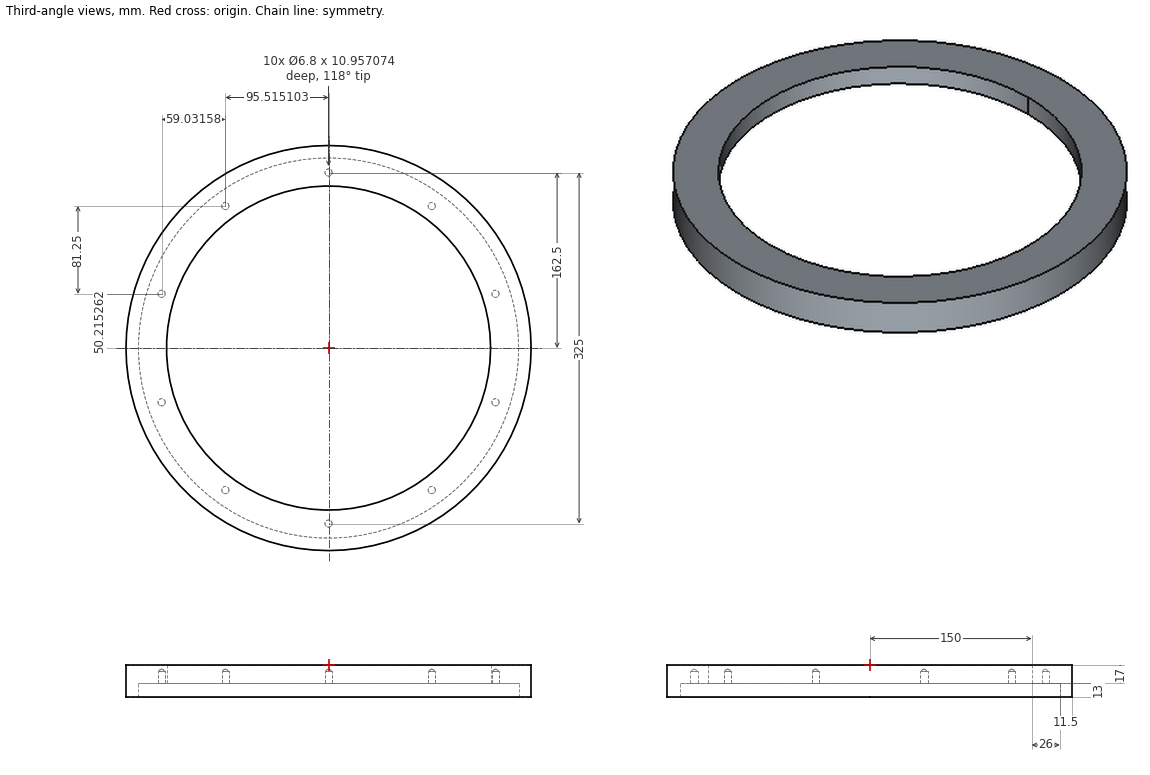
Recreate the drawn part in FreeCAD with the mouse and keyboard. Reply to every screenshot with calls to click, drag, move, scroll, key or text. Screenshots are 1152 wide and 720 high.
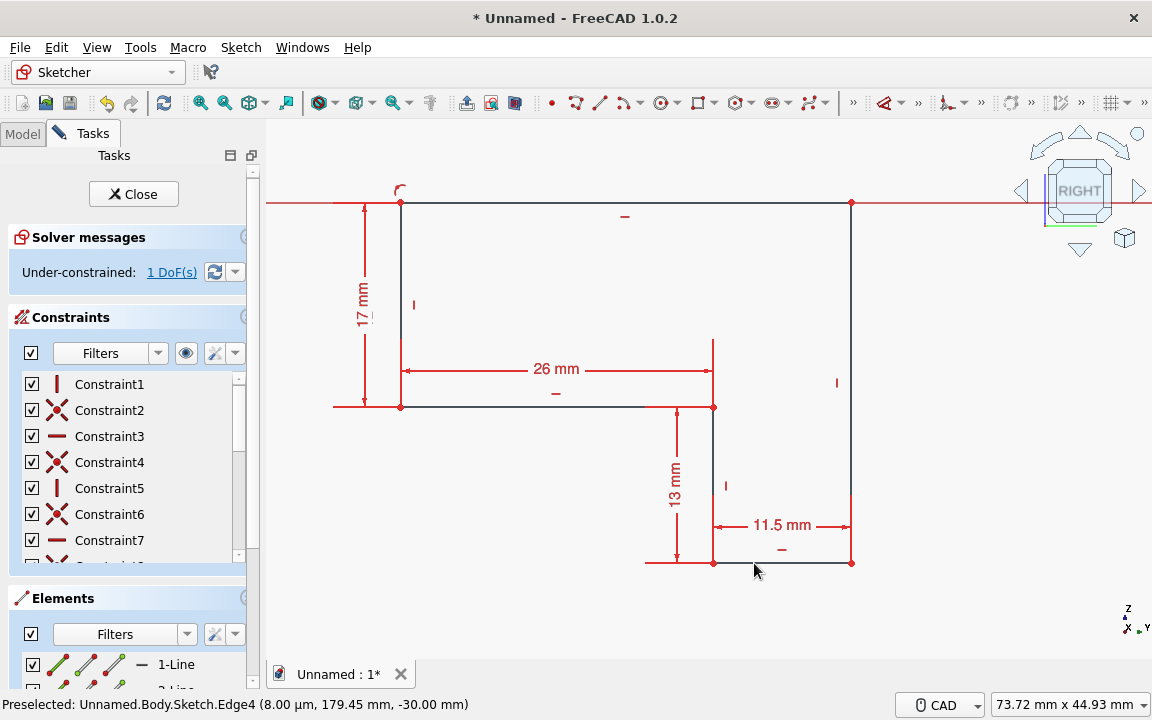
click(401, 203)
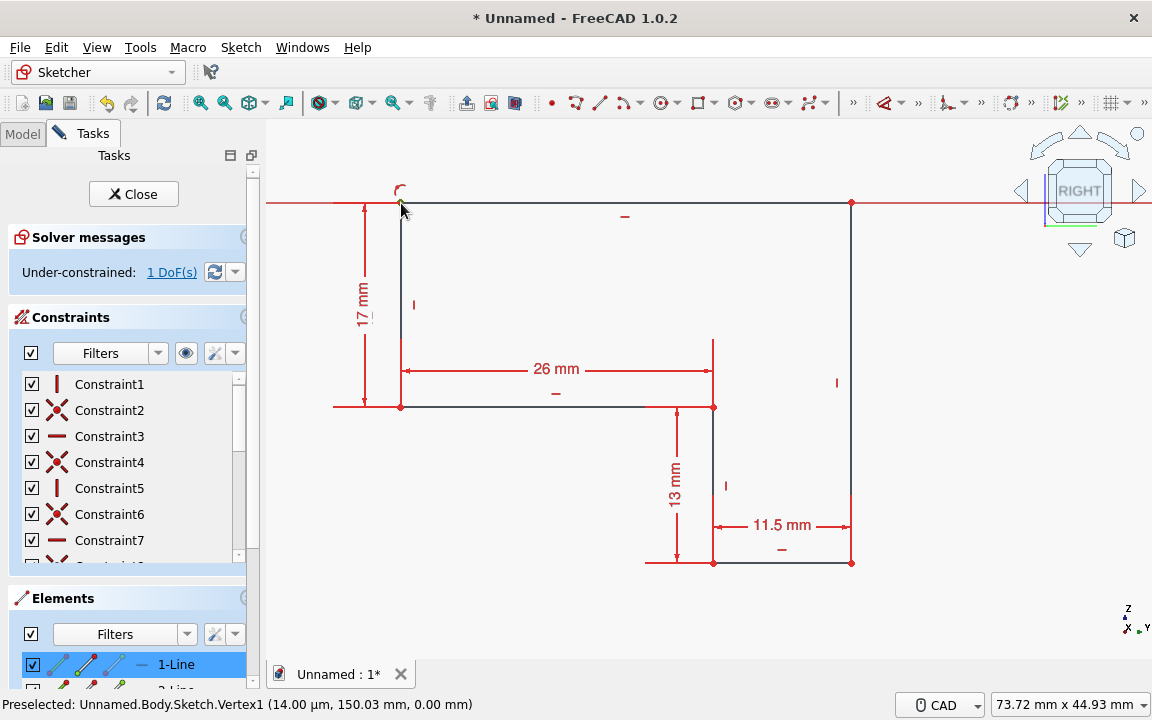
key(l)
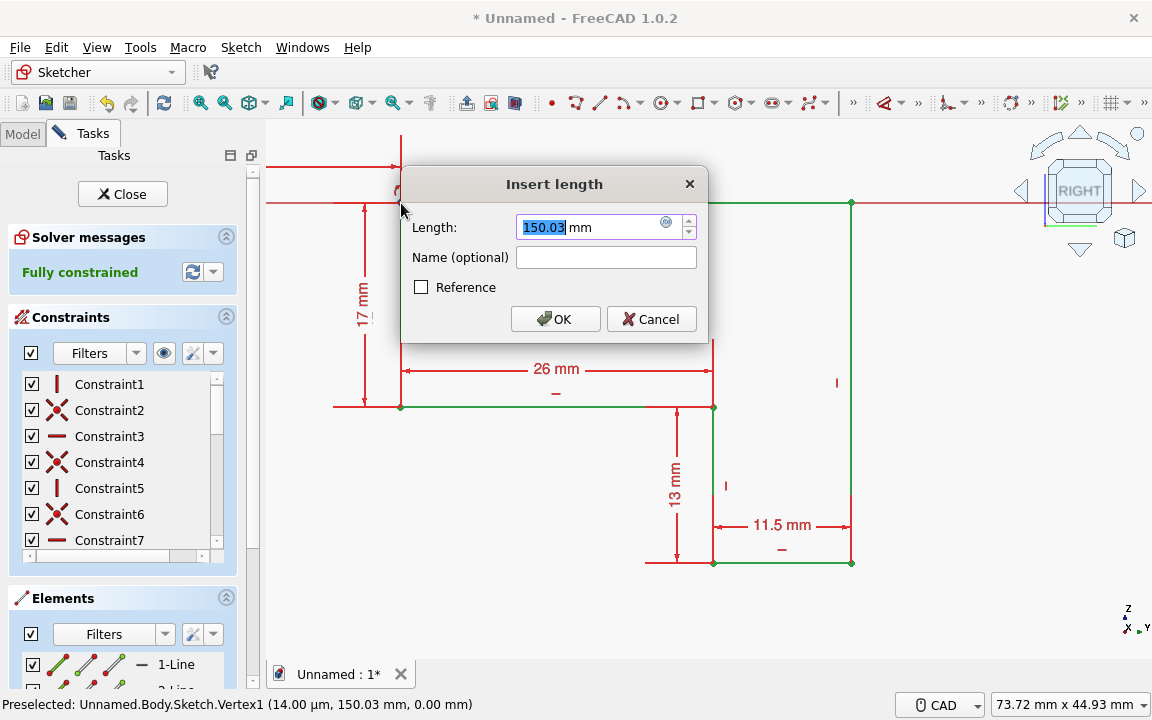
text(150)
key(Return)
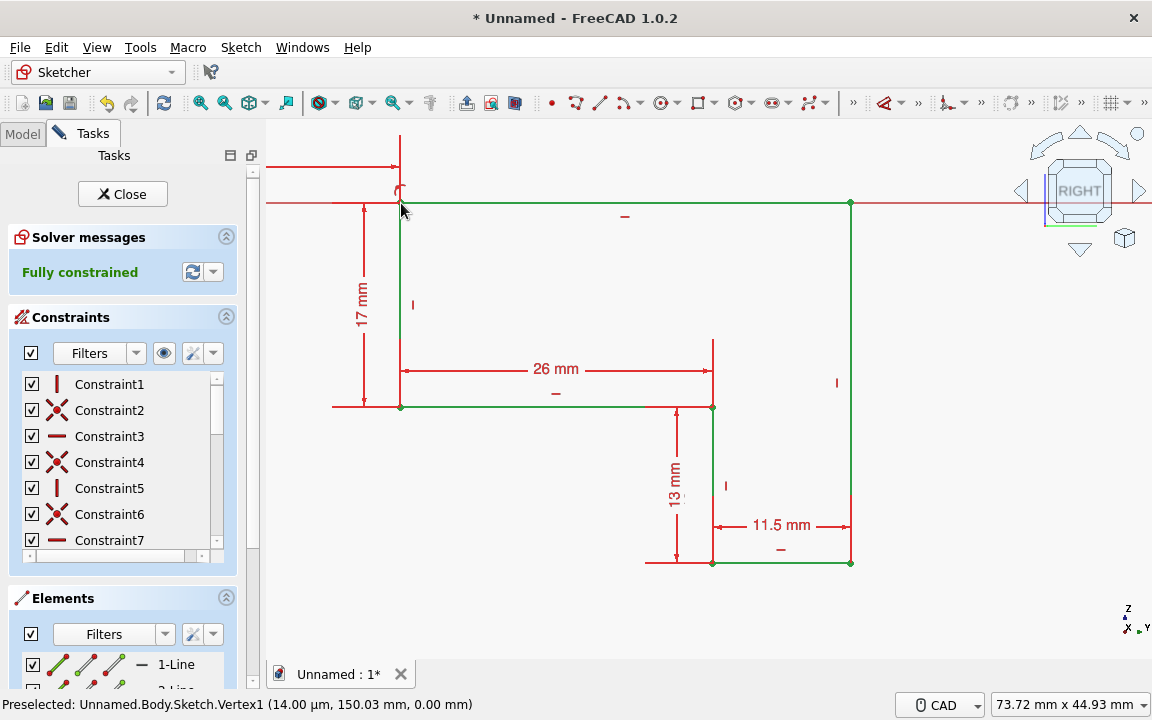
click(123, 194)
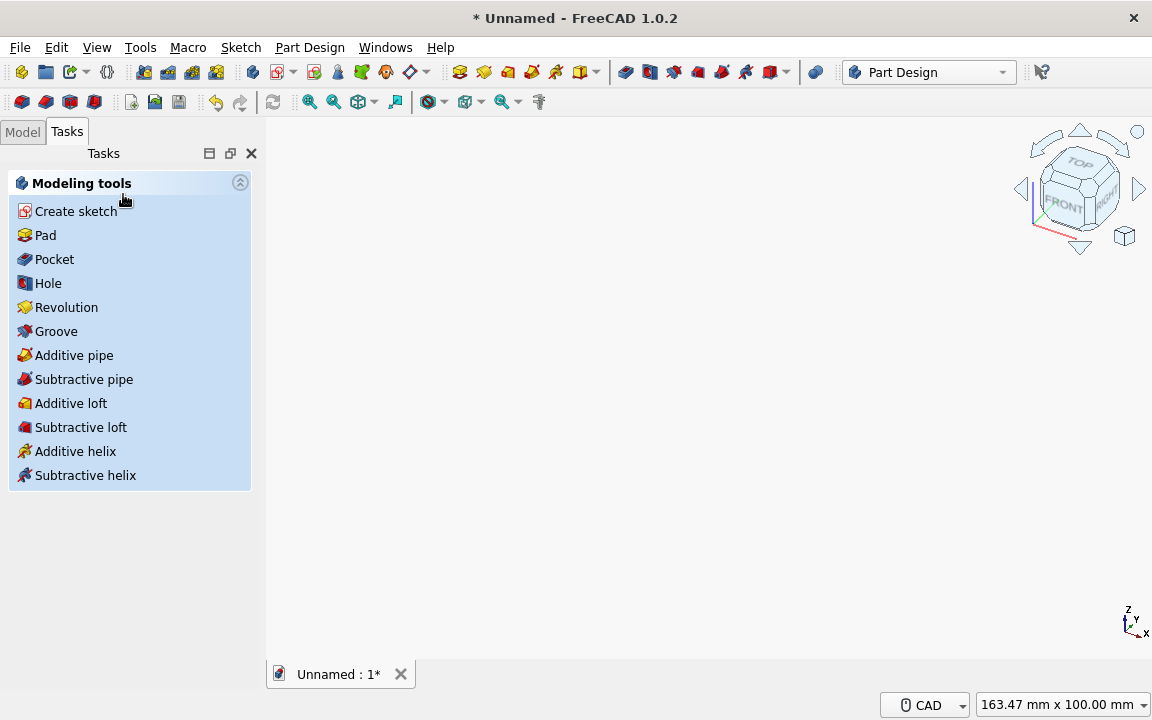
click(484, 72)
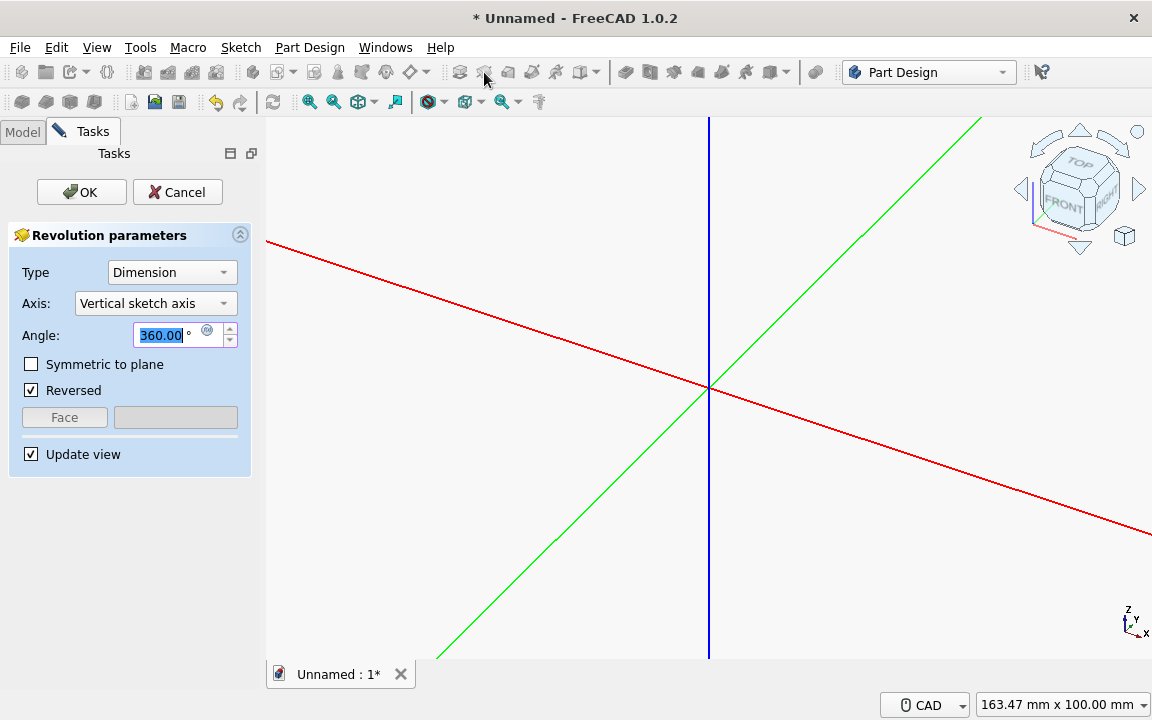
click(82, 192)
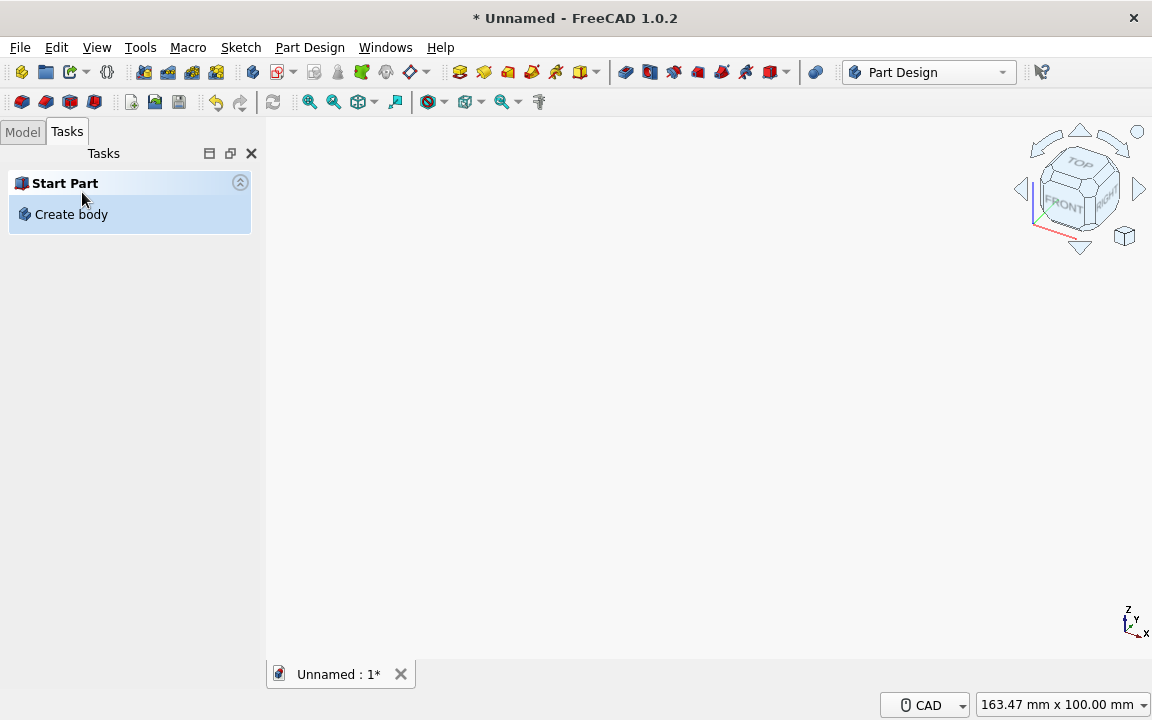
key(v)
key(f)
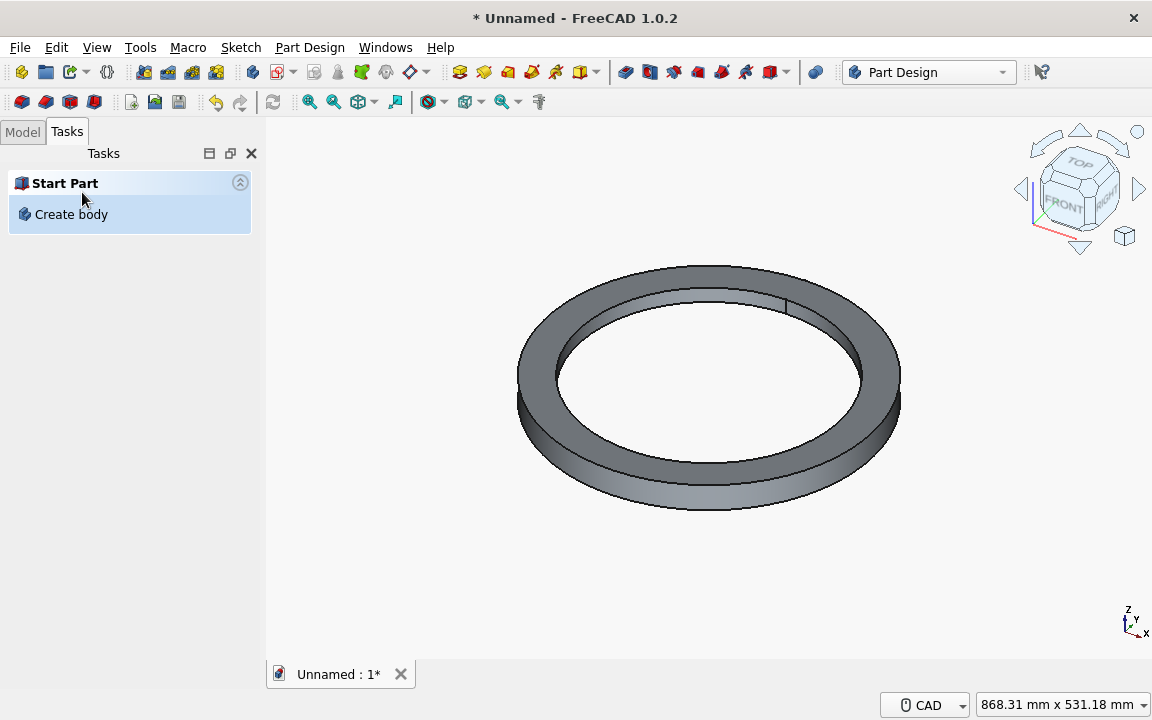
key(5)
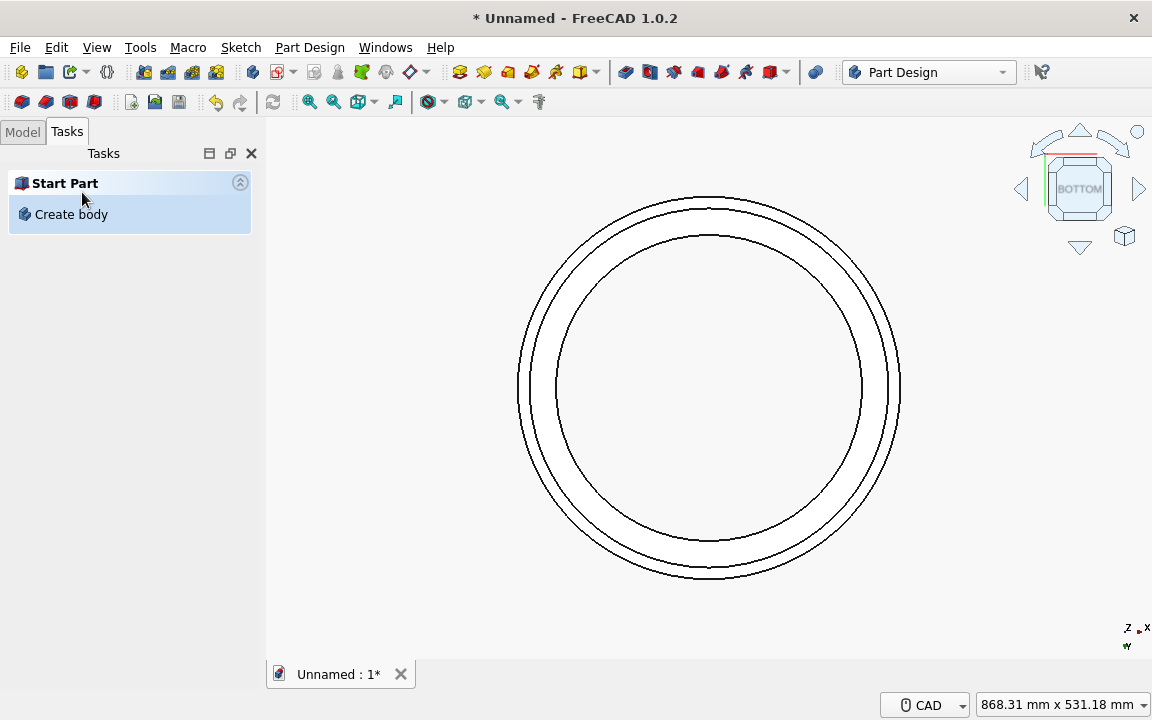
click(658, 233)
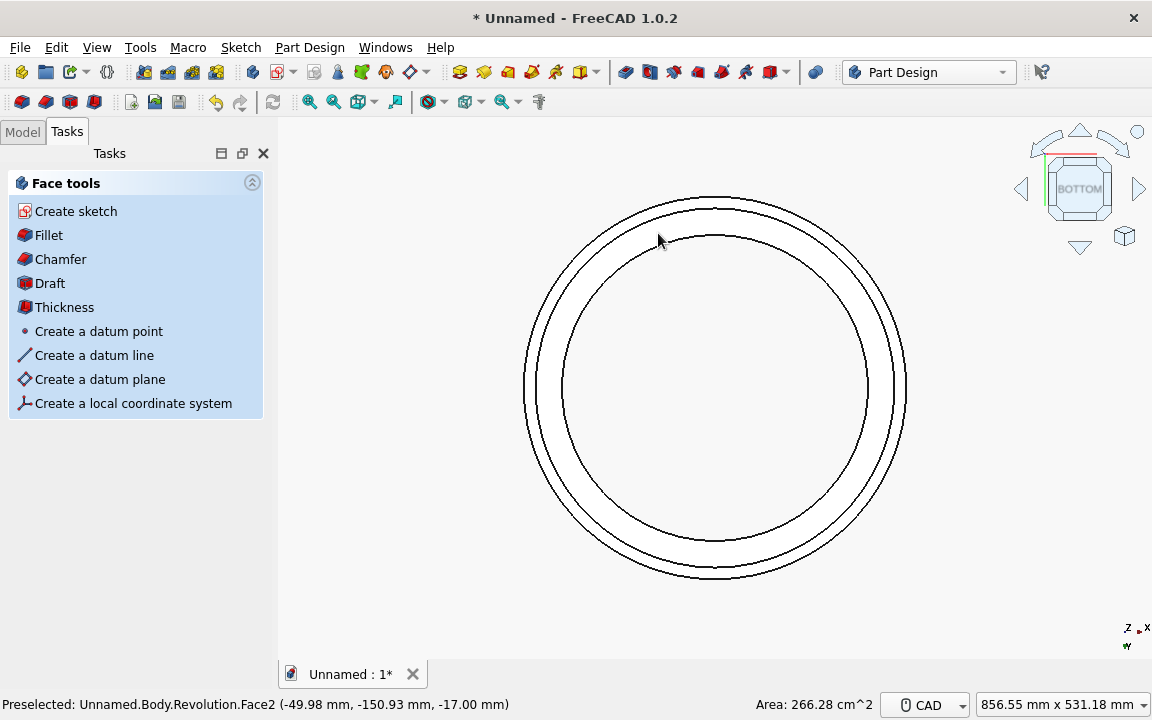
click(278, 72)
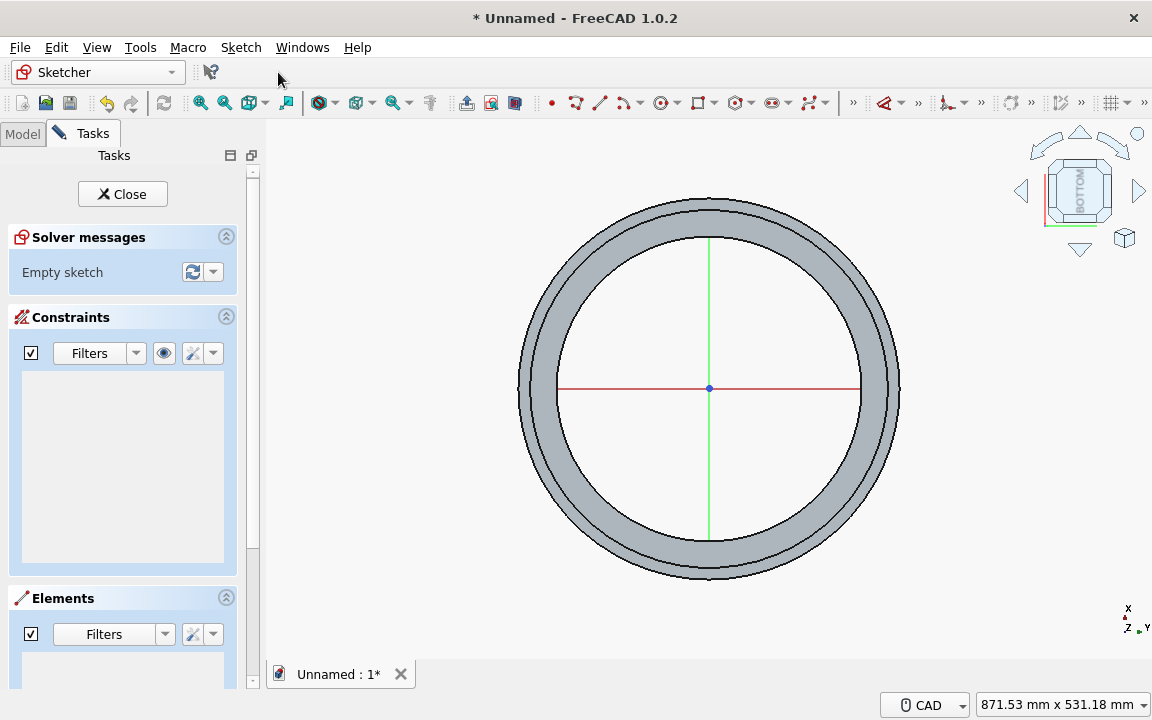
click(662, 104)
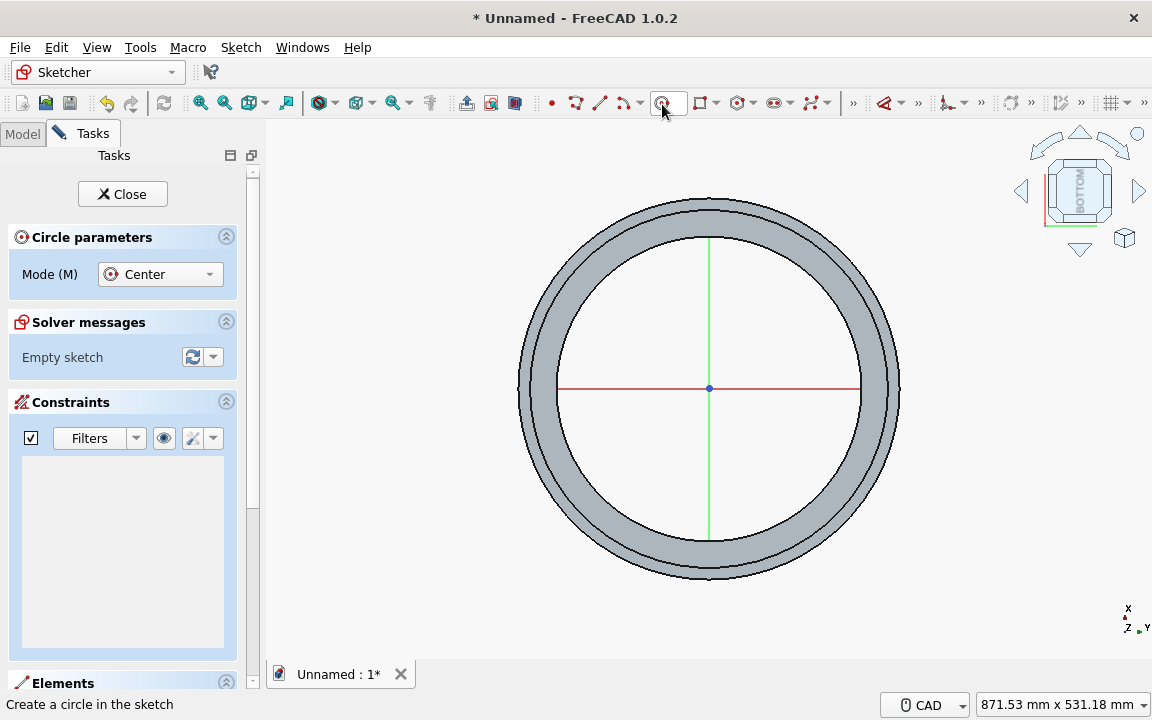
scroll(874, 389, up, 10)